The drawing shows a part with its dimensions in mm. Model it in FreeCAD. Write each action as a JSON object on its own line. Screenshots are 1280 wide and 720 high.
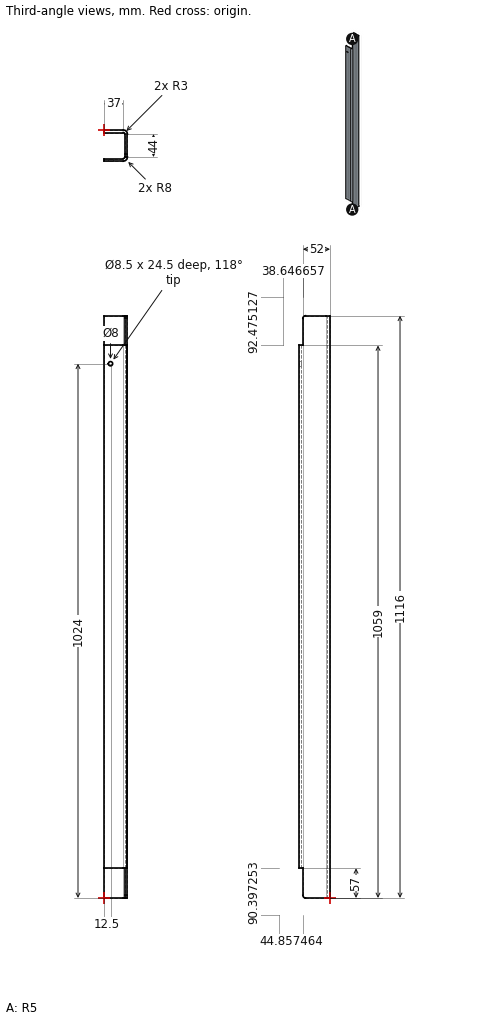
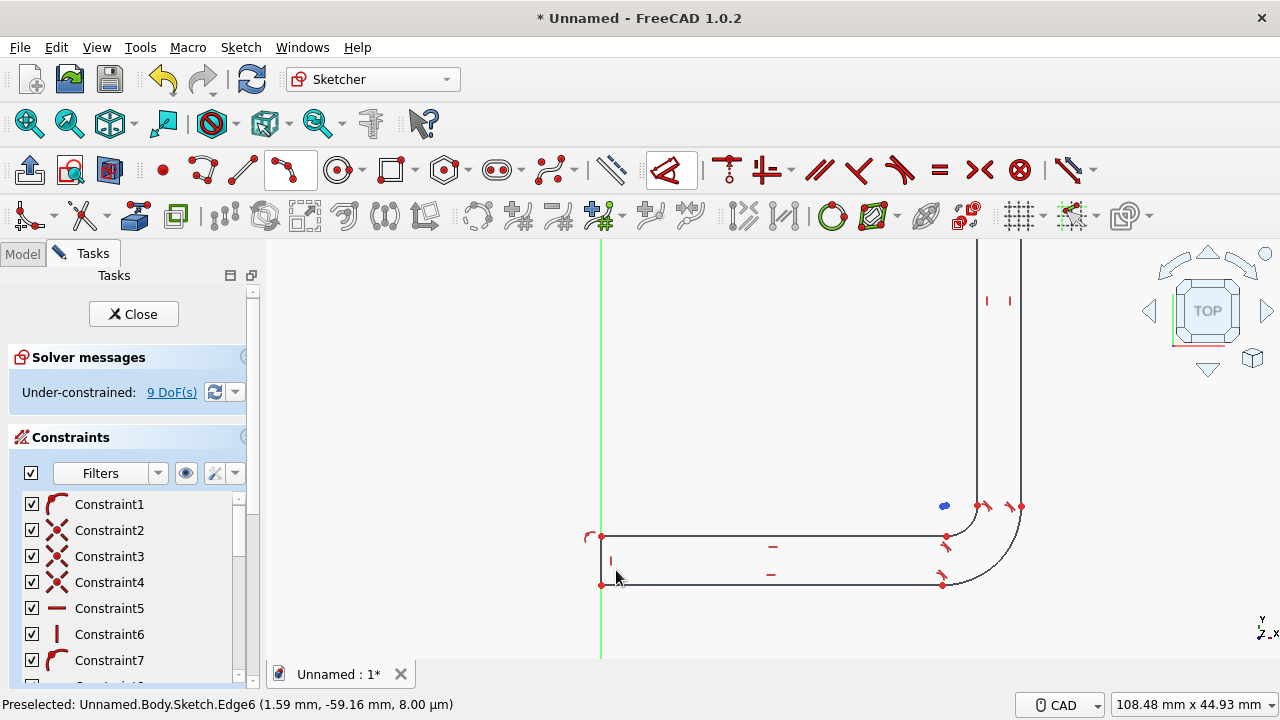
{"action": "left_click", "coordinate": [961, 533]}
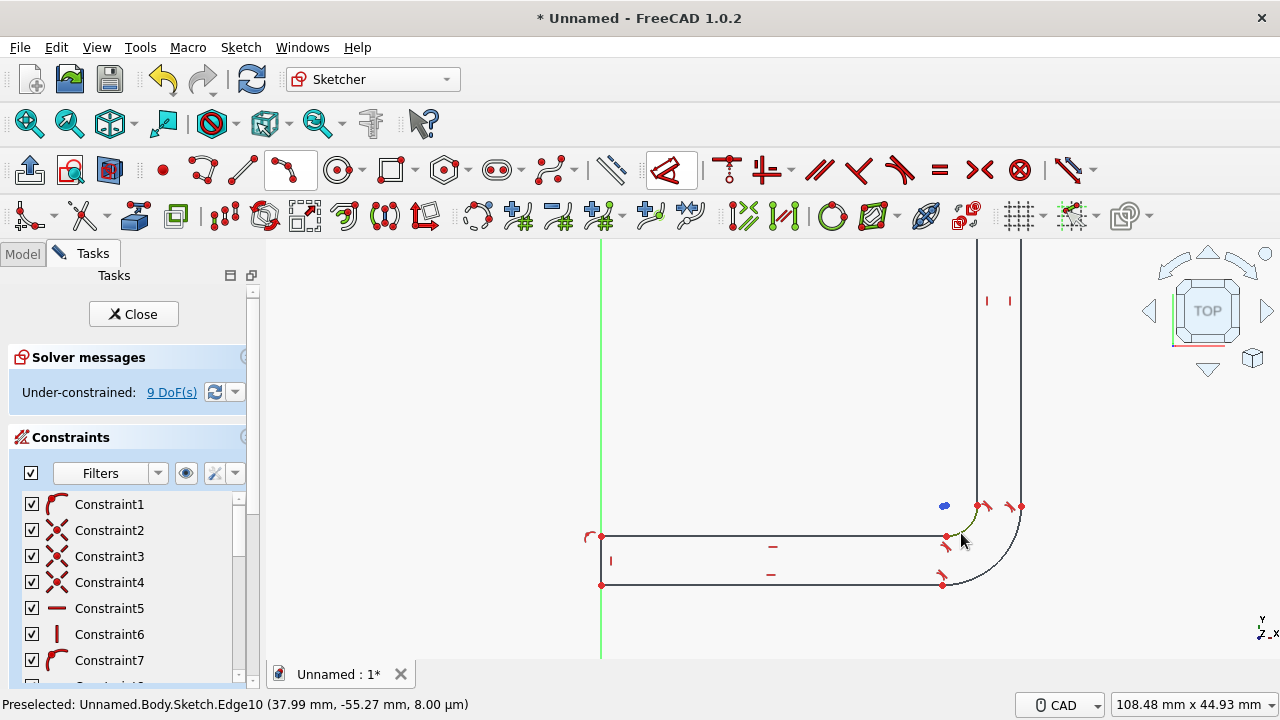
{"action": "left_click", "coordinate": [978, 577]}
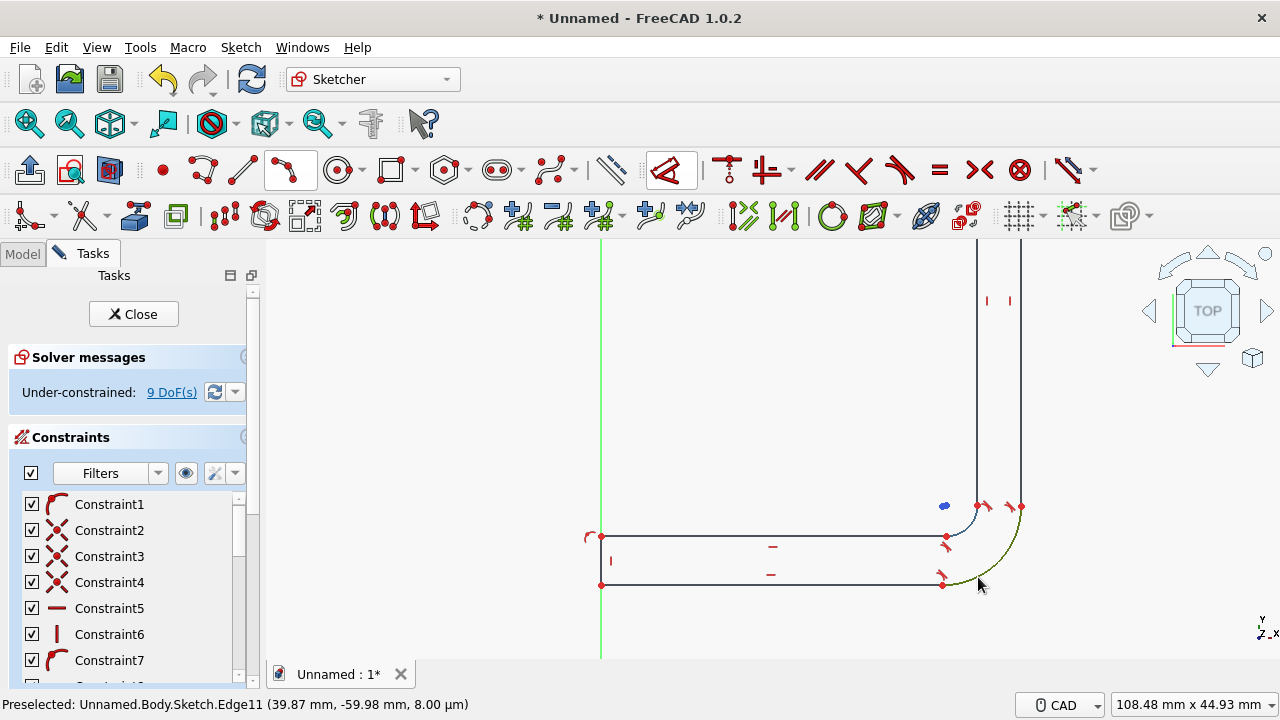
{"action": "left_click", "coordinate": [728, 170]}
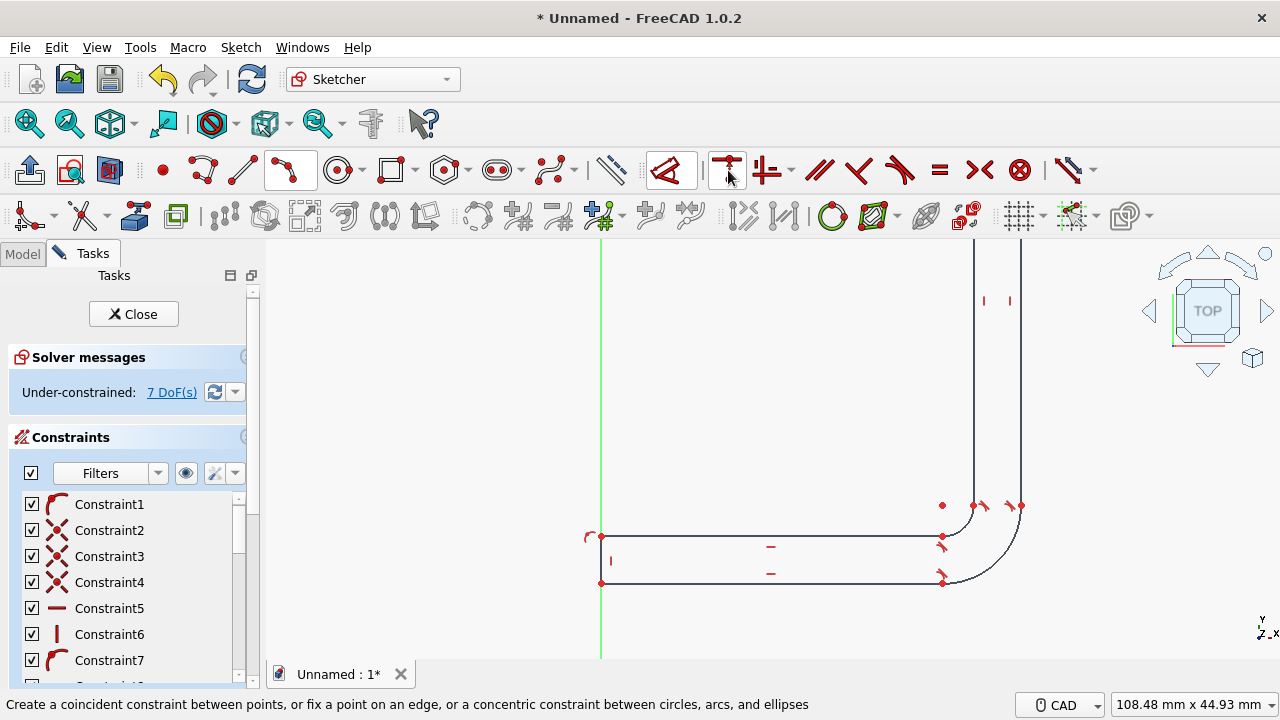
{"action": "scroll", "coordinate": [617, 572], "scroll_direction": "down", "scroll_amount": 4}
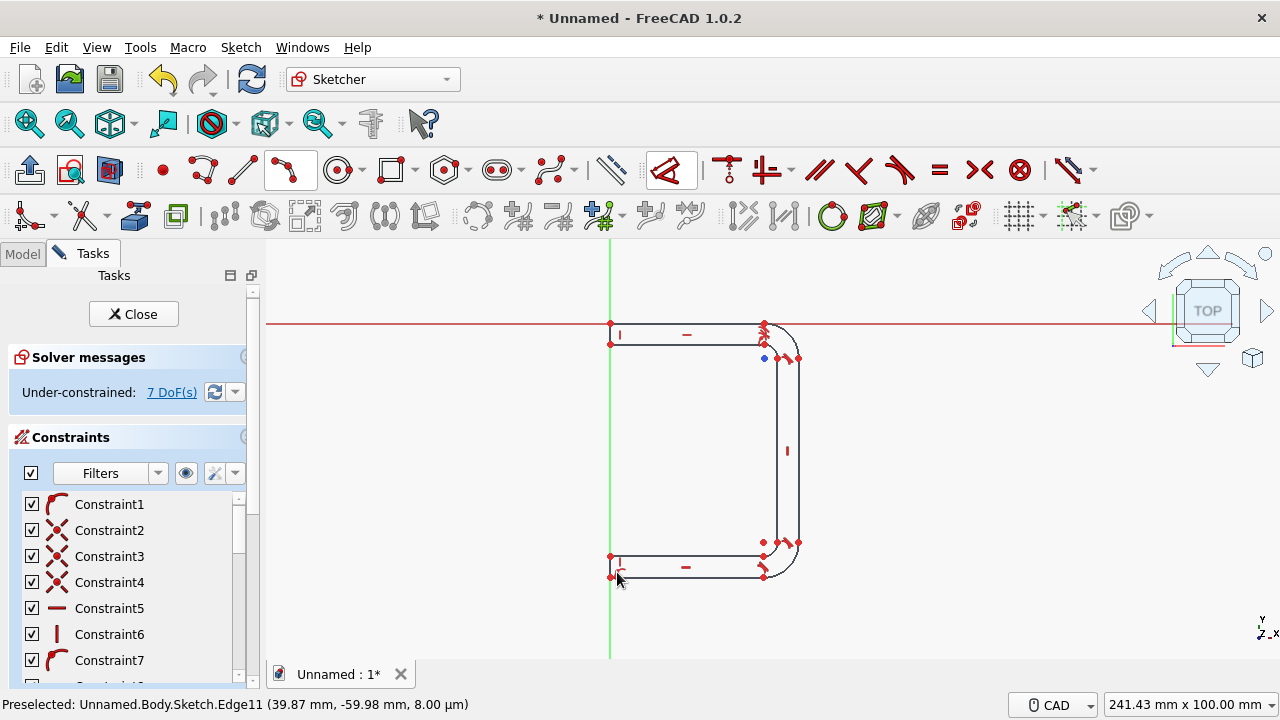
{"action": "scroll", "coordinate": [776, 352], "scroll_direction": "up", "scroll_amount": 4}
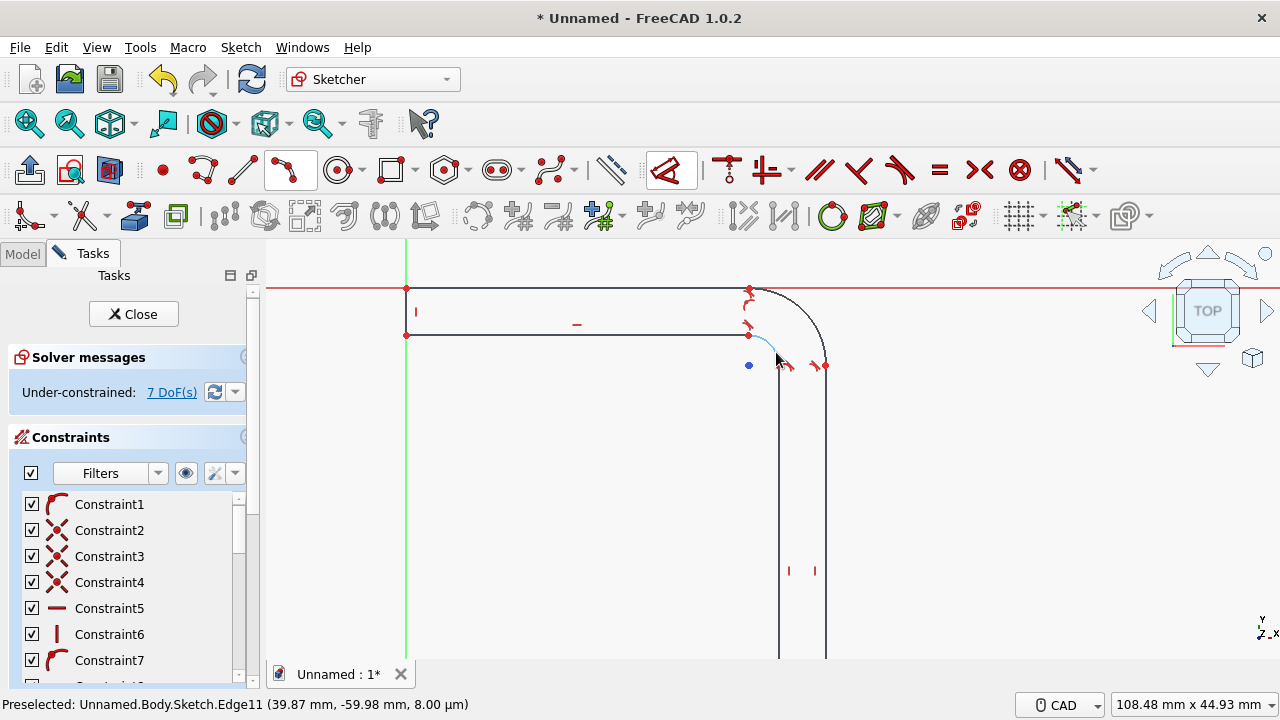
{"action": "left_click", "coordinate": [775, 352]}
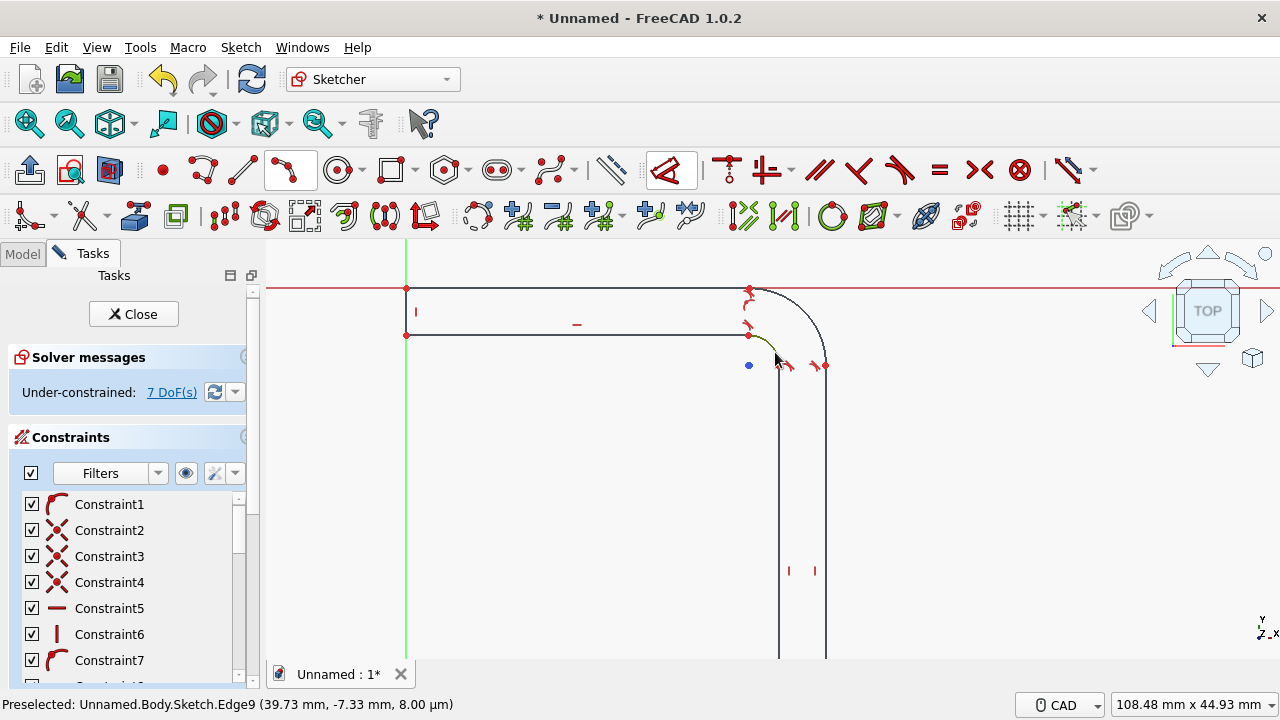
{"action": "left_click", "coordinate": [818, 330]}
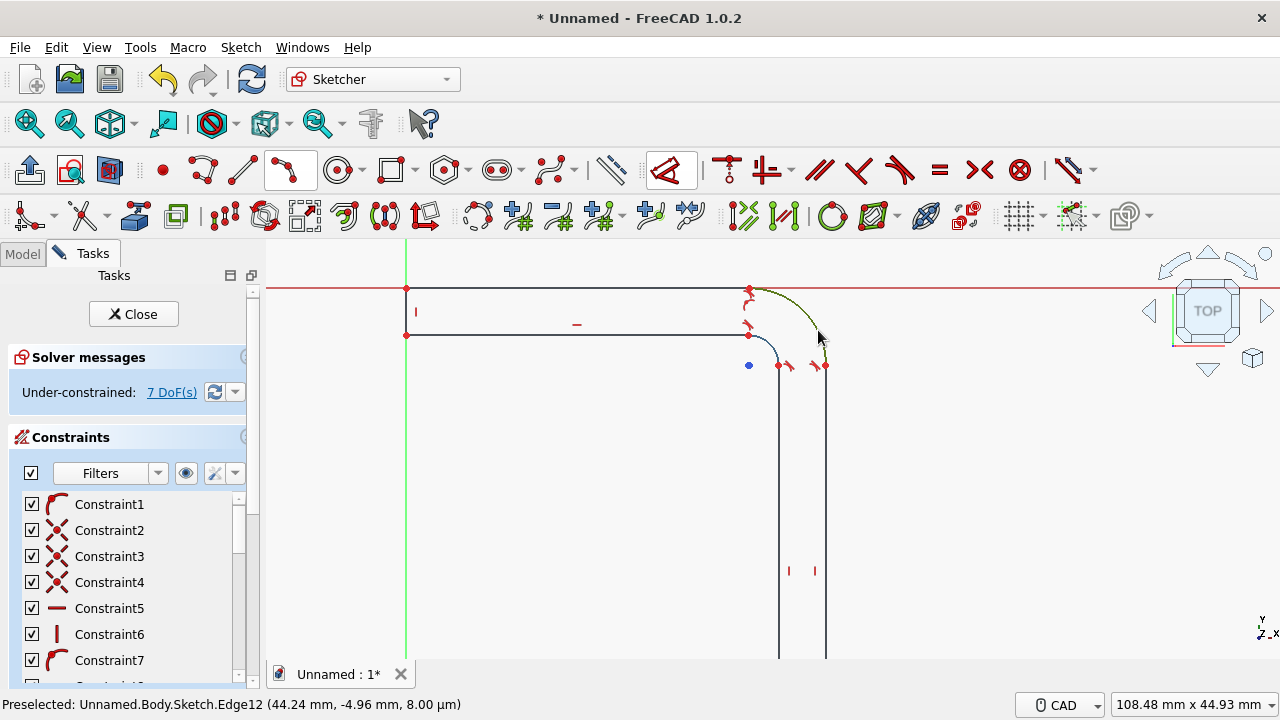
{"action": "left_click", "coordinate": [728, 170]}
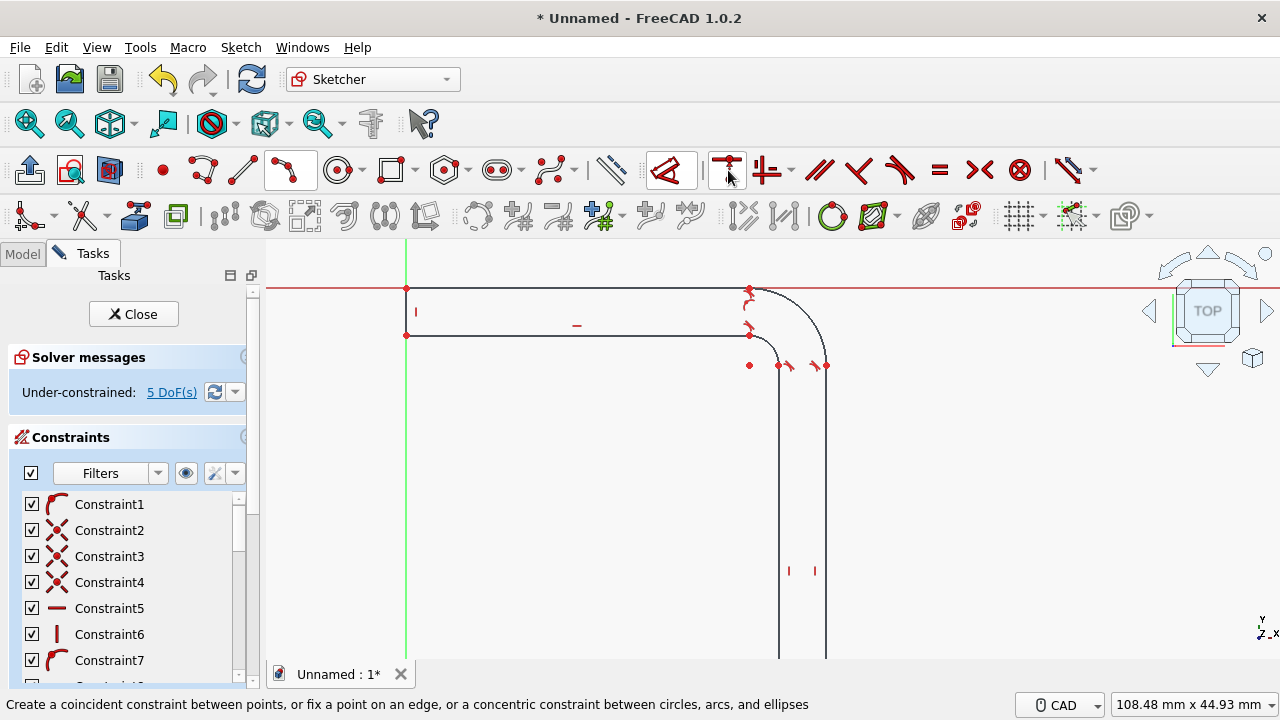
{"action": "left_click", "coordinate": [776, 352]}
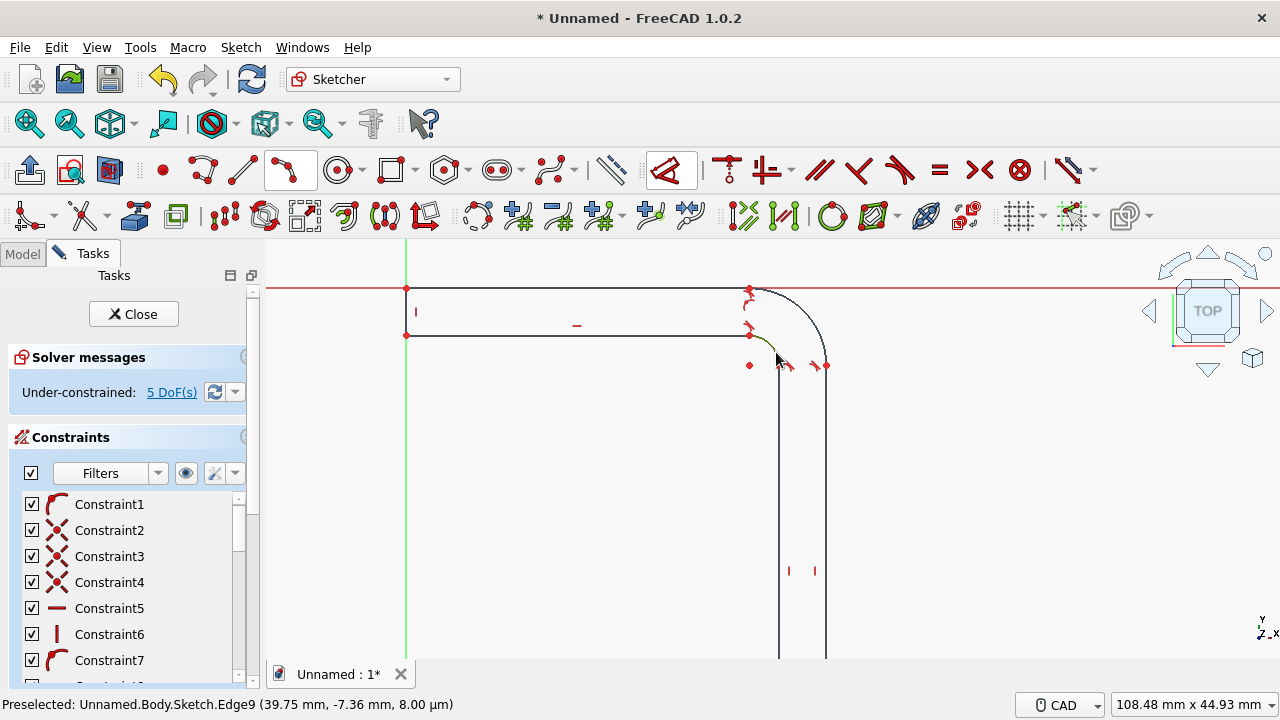
{"action": "scroll", "coordinate": [776, 351], "scroll_direction": "down", "scroll_amount": 4}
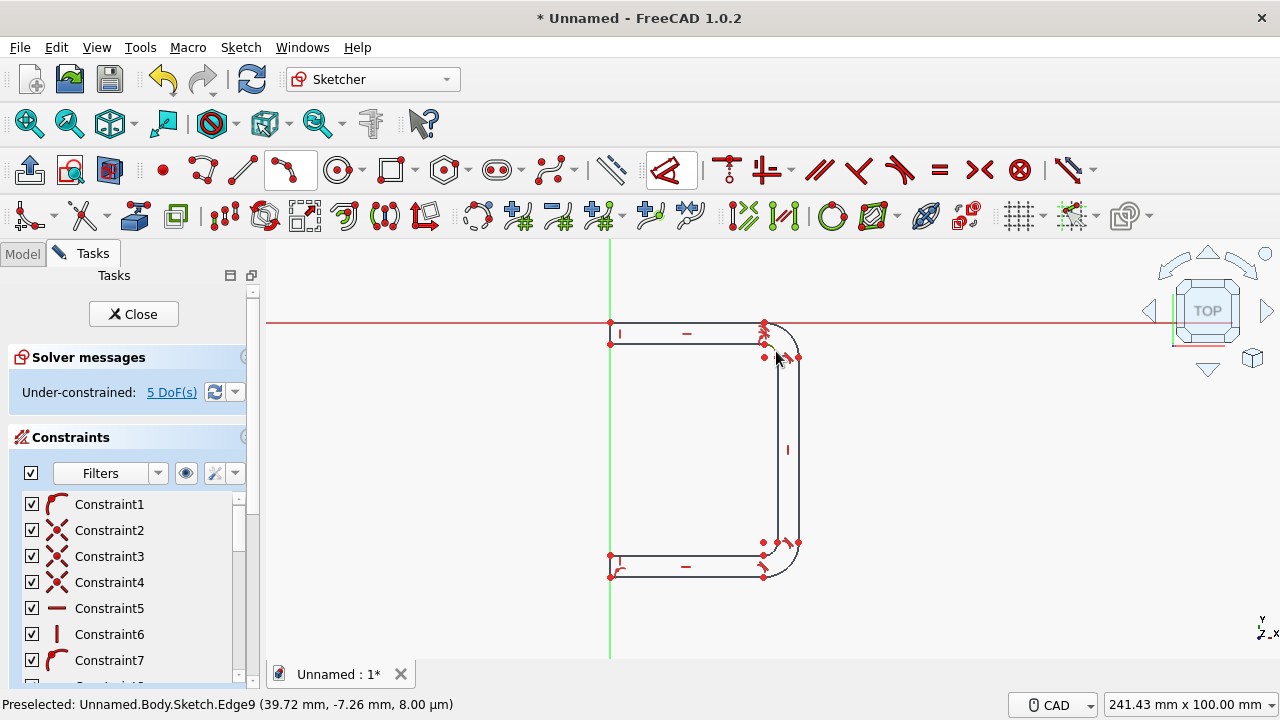
{"action": "scroll", "coordinate": [770, 554], "scroll_direction": "up", "scroll_amount": 4}